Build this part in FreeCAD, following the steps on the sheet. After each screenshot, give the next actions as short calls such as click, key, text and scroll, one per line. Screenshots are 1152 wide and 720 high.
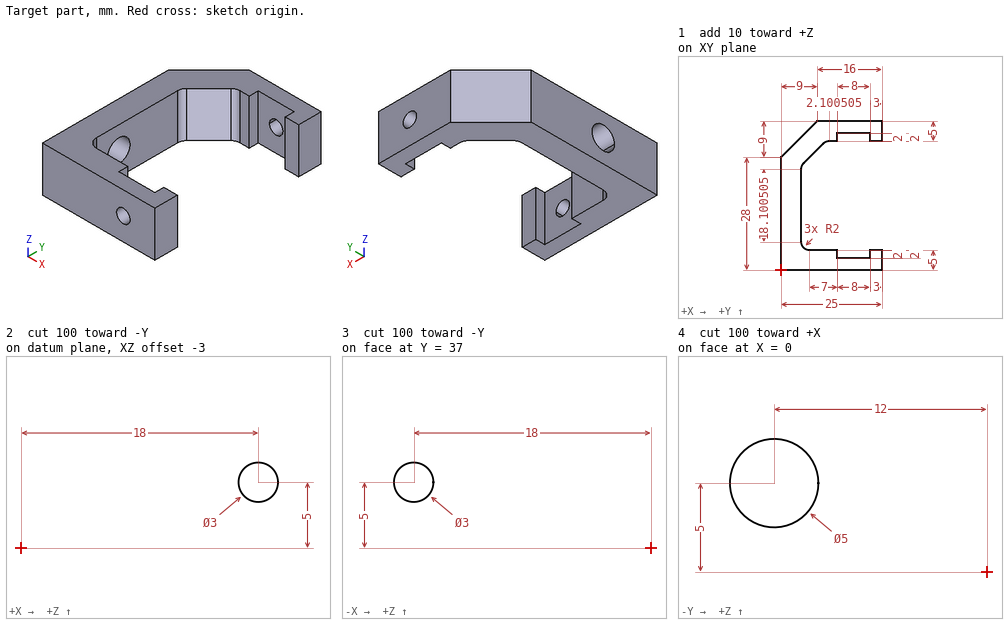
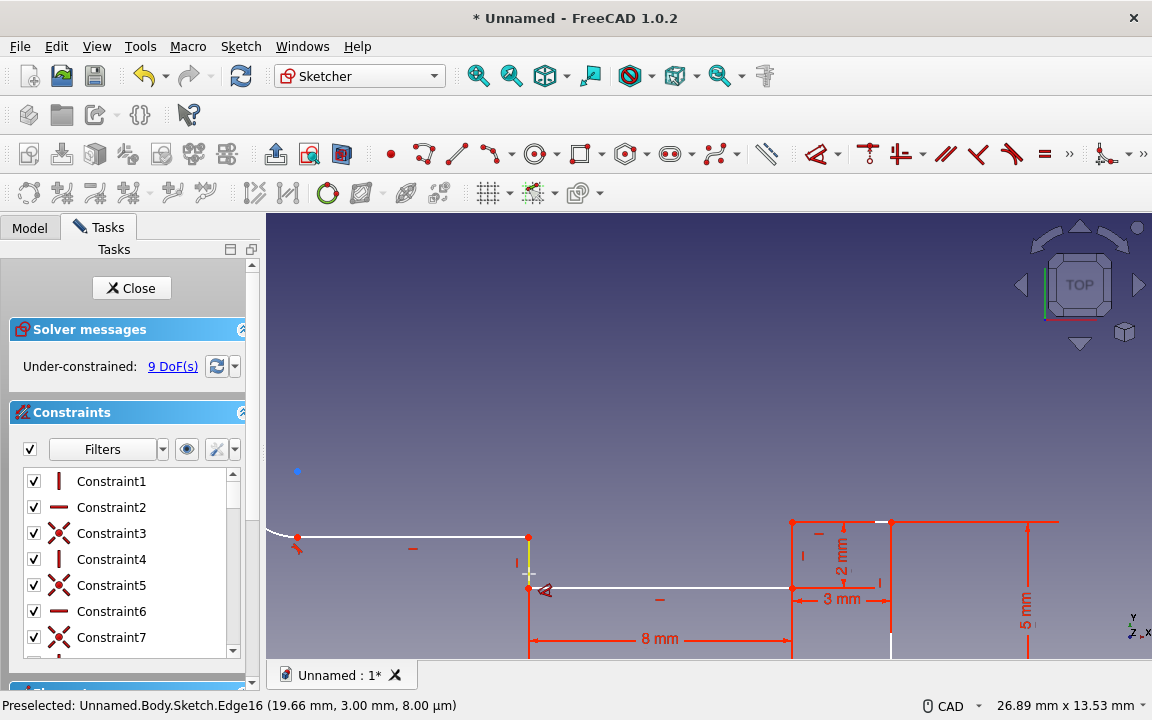
click(529, 573)
click(563, 563)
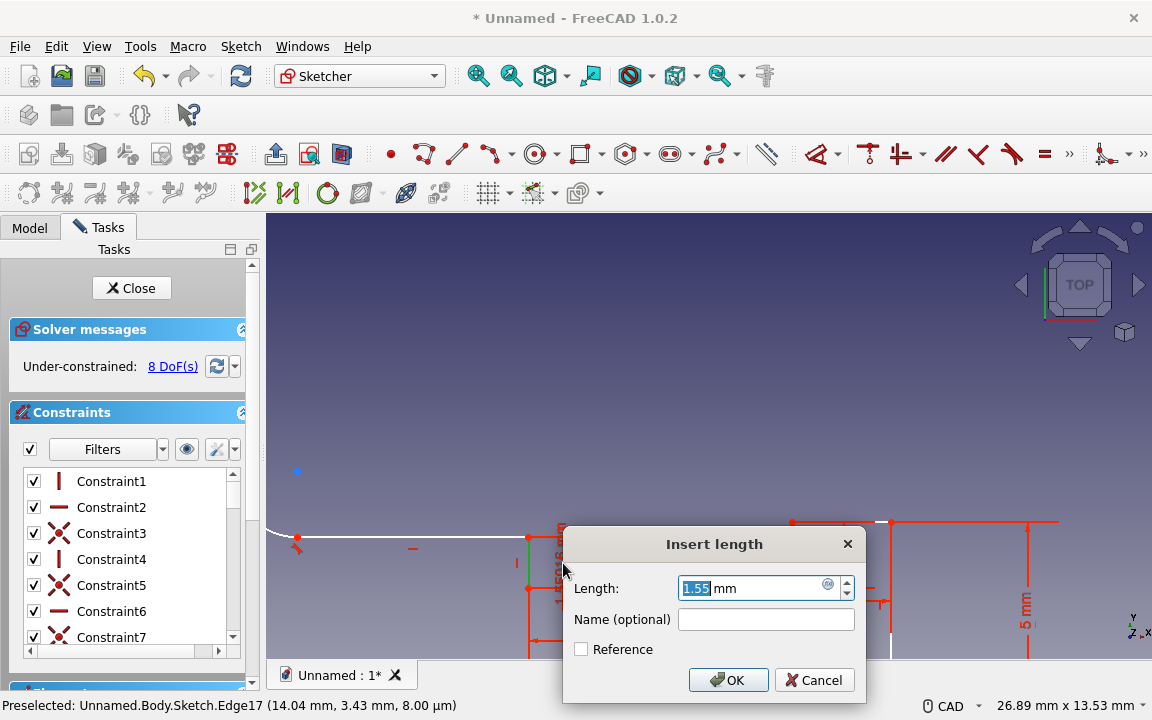
text(2)
key(Return)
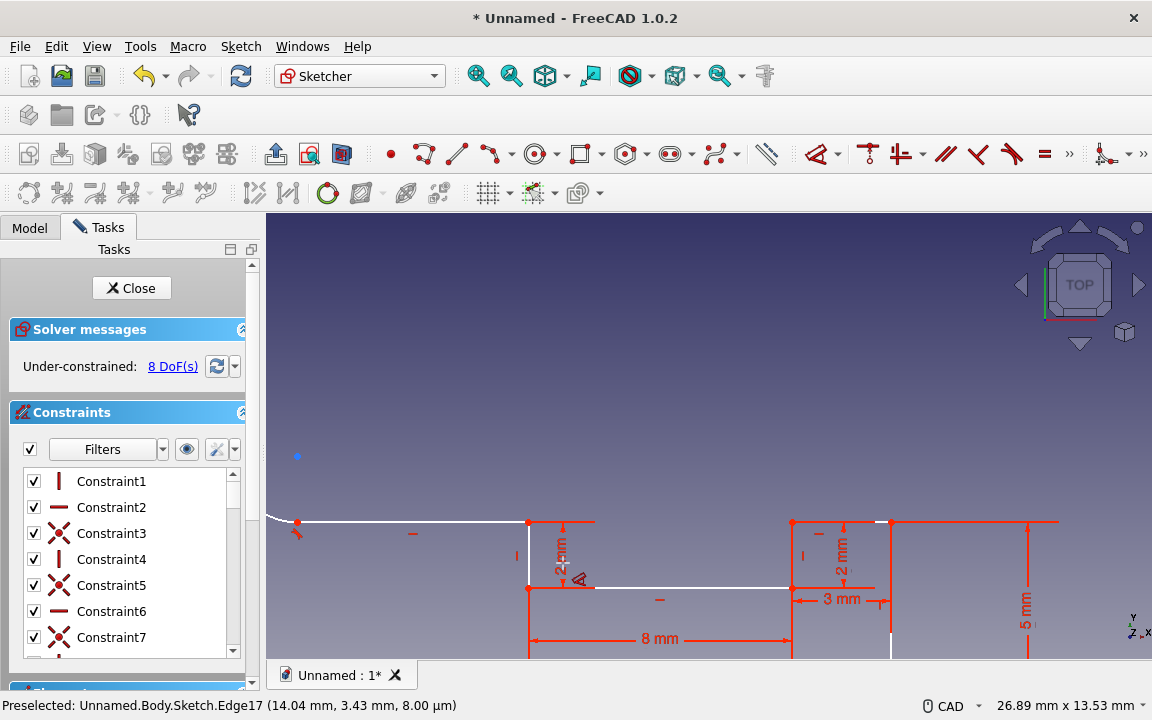
scroll(694, 553, down, 7)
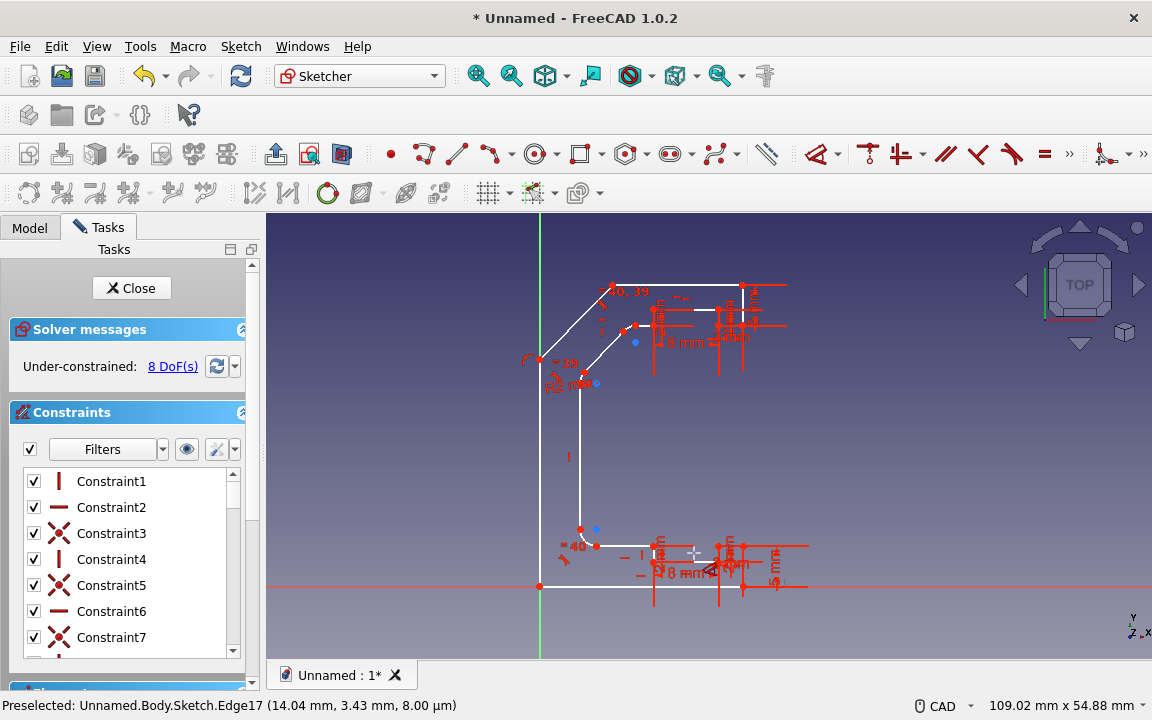
click(637, 546)
click(625, 512)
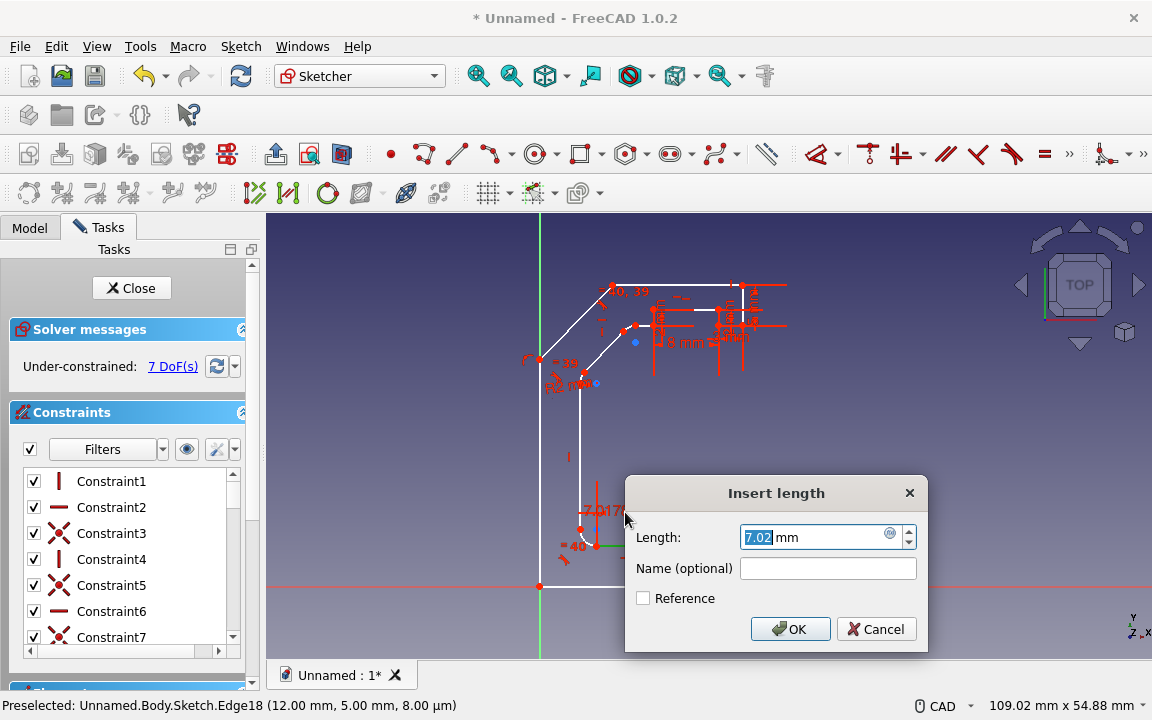
text(7)
key(Return)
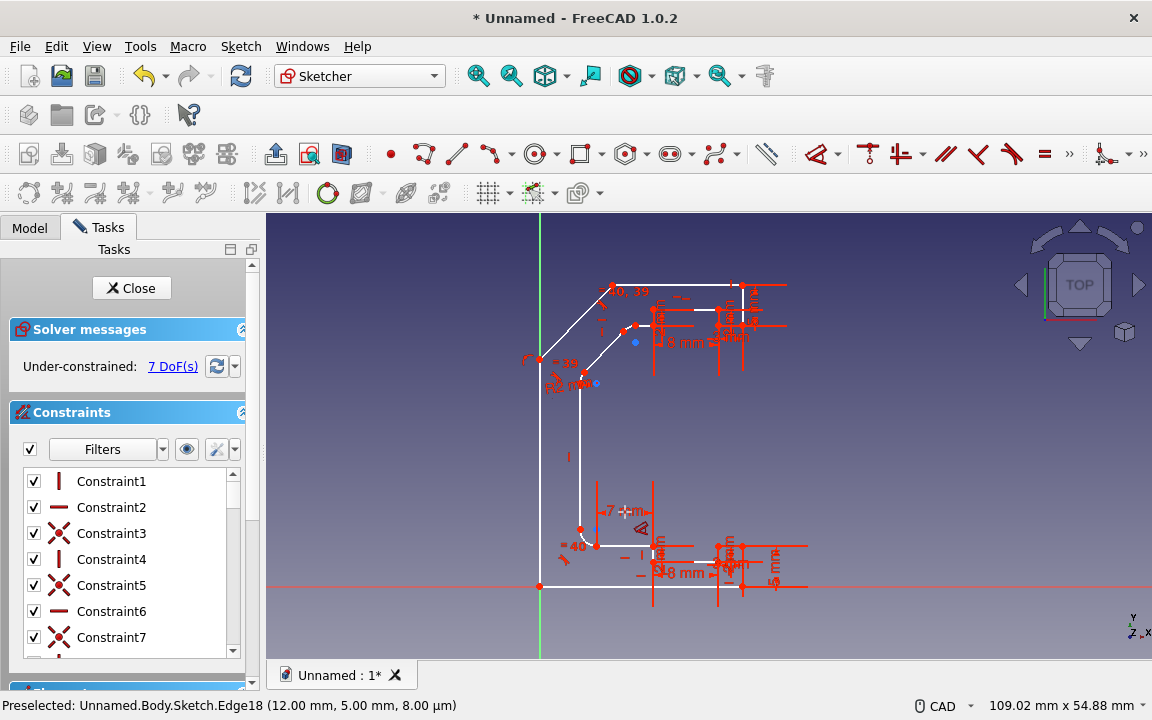
click(704, 285)
click(678, 251)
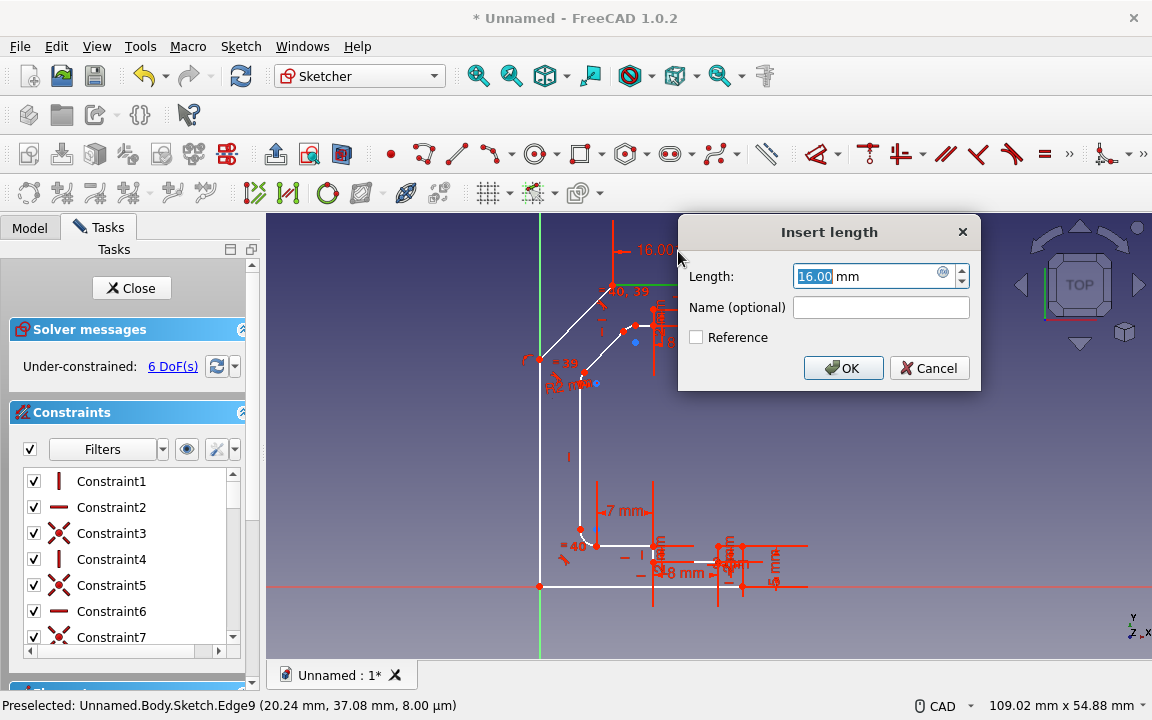
text(16)
key(Return)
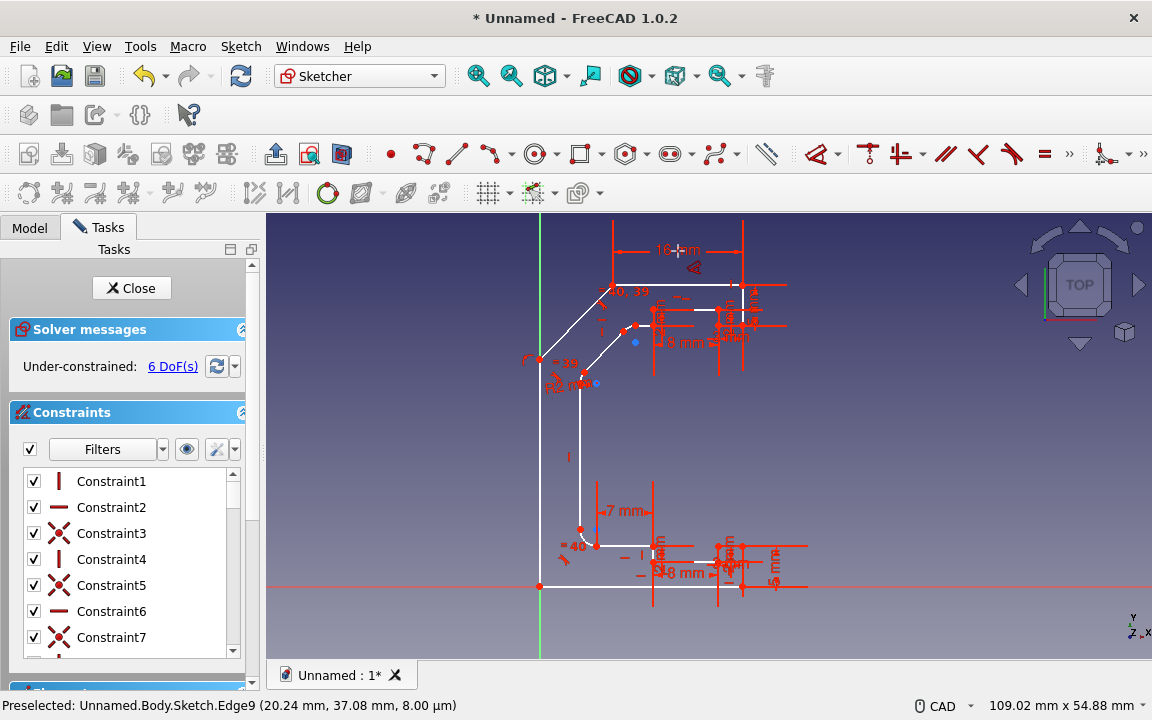
click(540, 428)
click(506, 473)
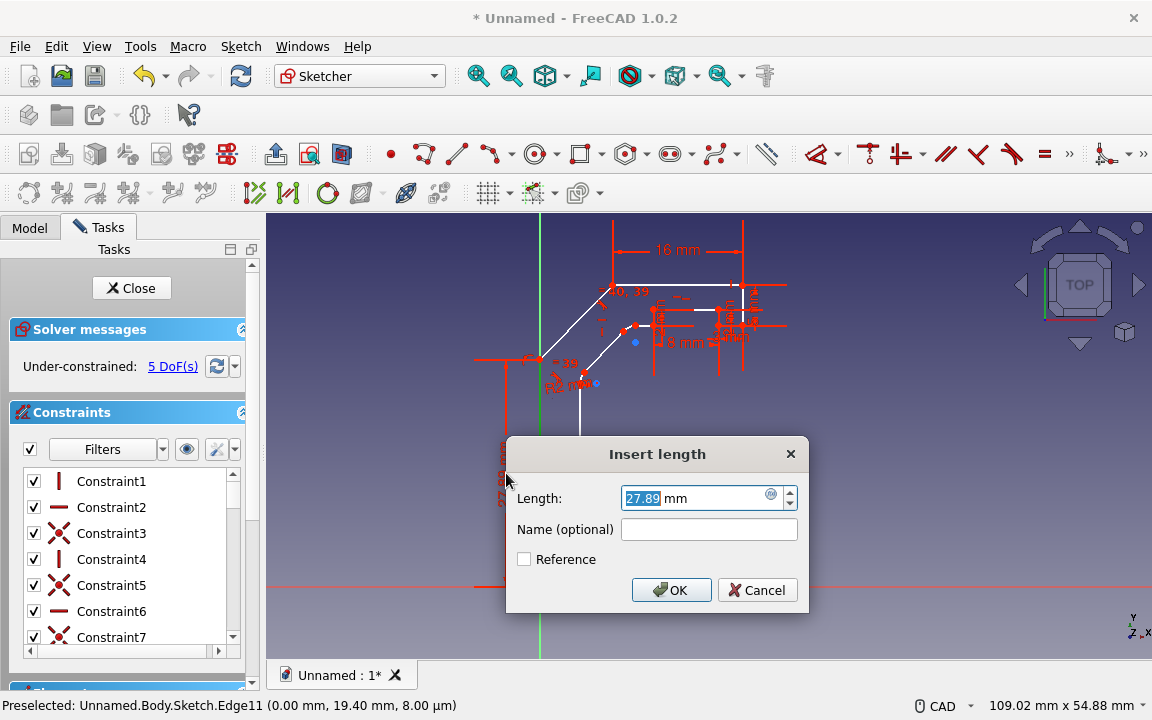
text(28)
key(Return)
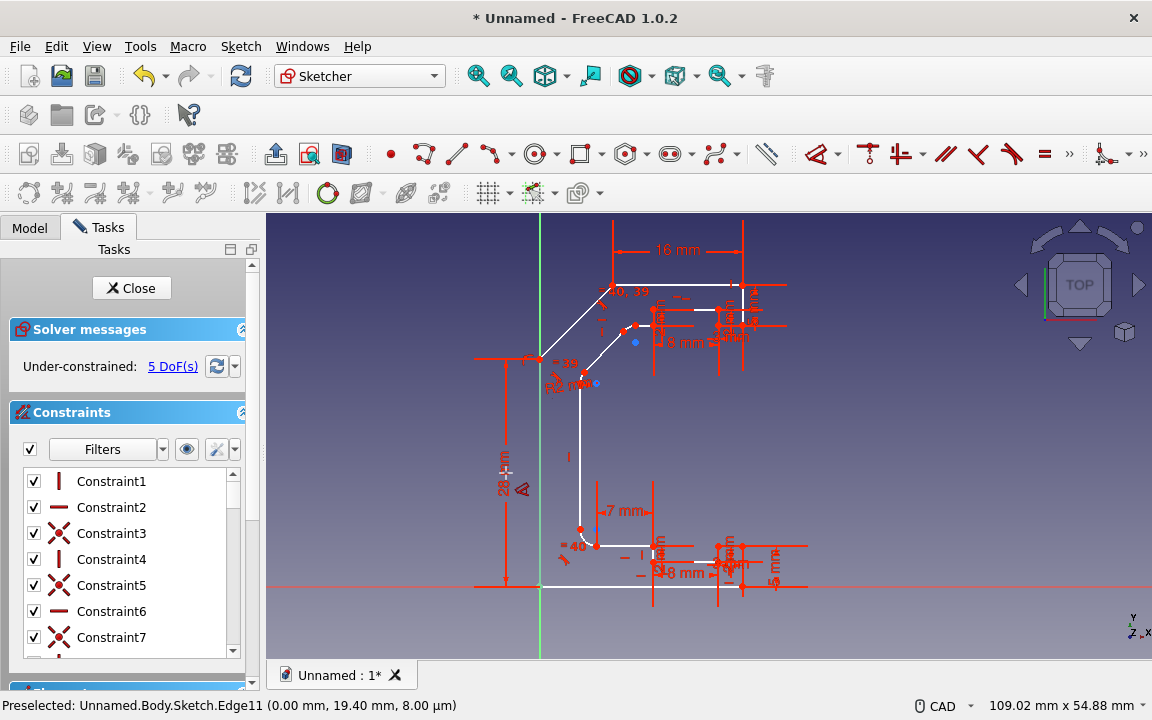
click(601, 587)
click(641, 621)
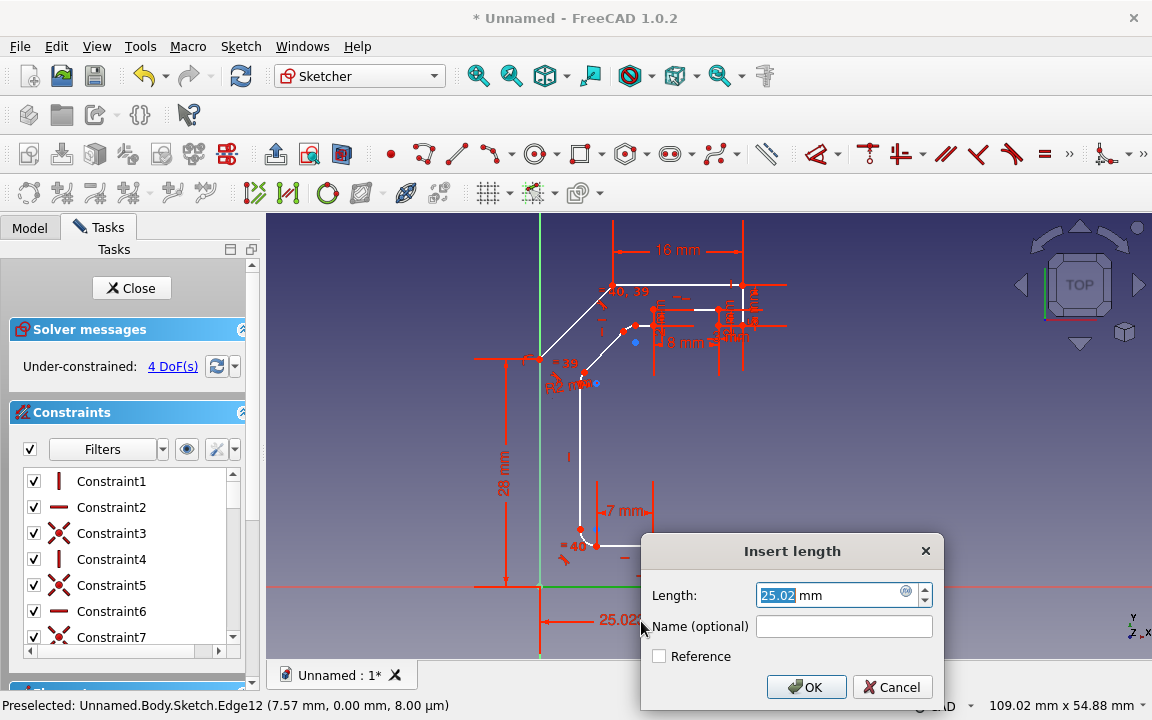
text(25)
key(Return)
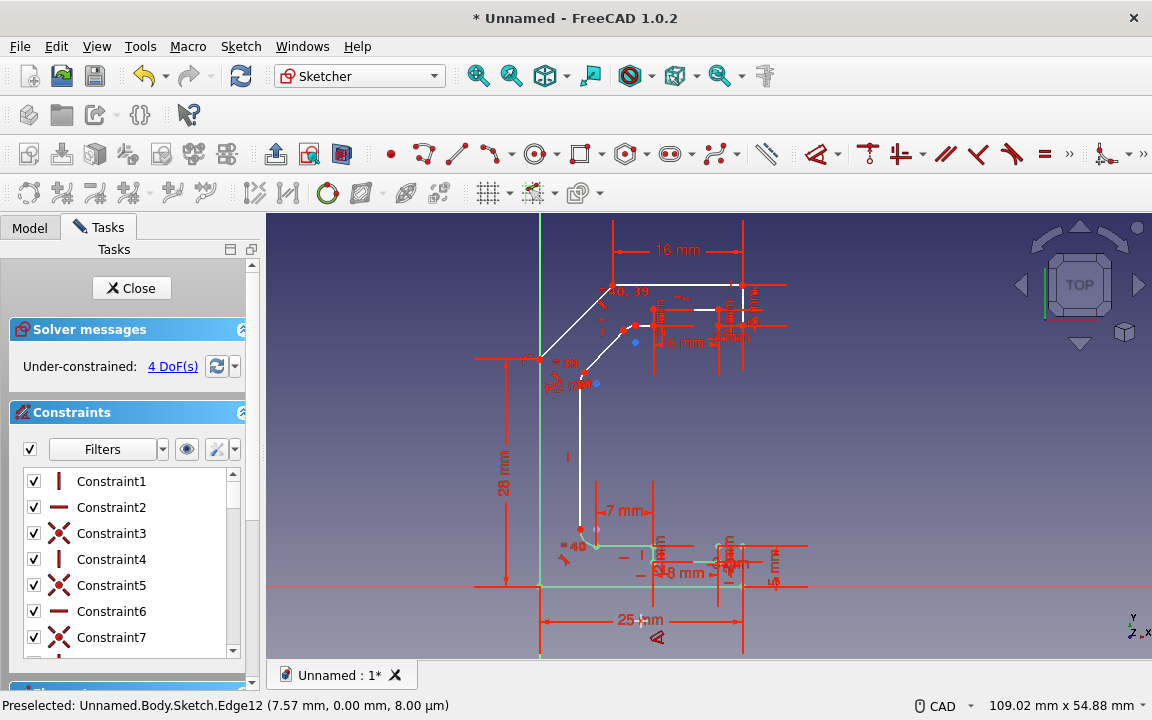
click(613, 285)
click(576, 251)